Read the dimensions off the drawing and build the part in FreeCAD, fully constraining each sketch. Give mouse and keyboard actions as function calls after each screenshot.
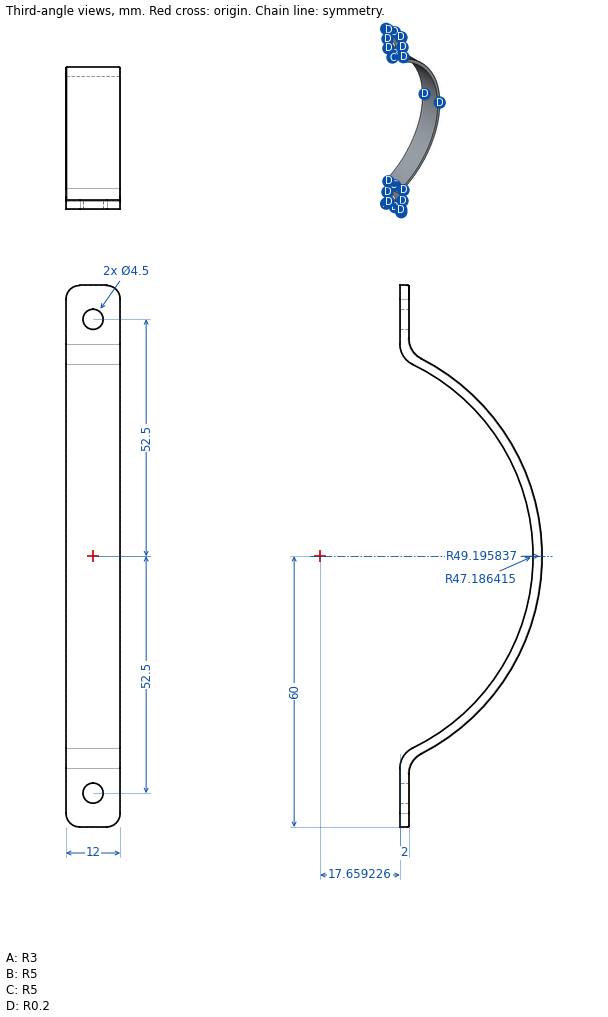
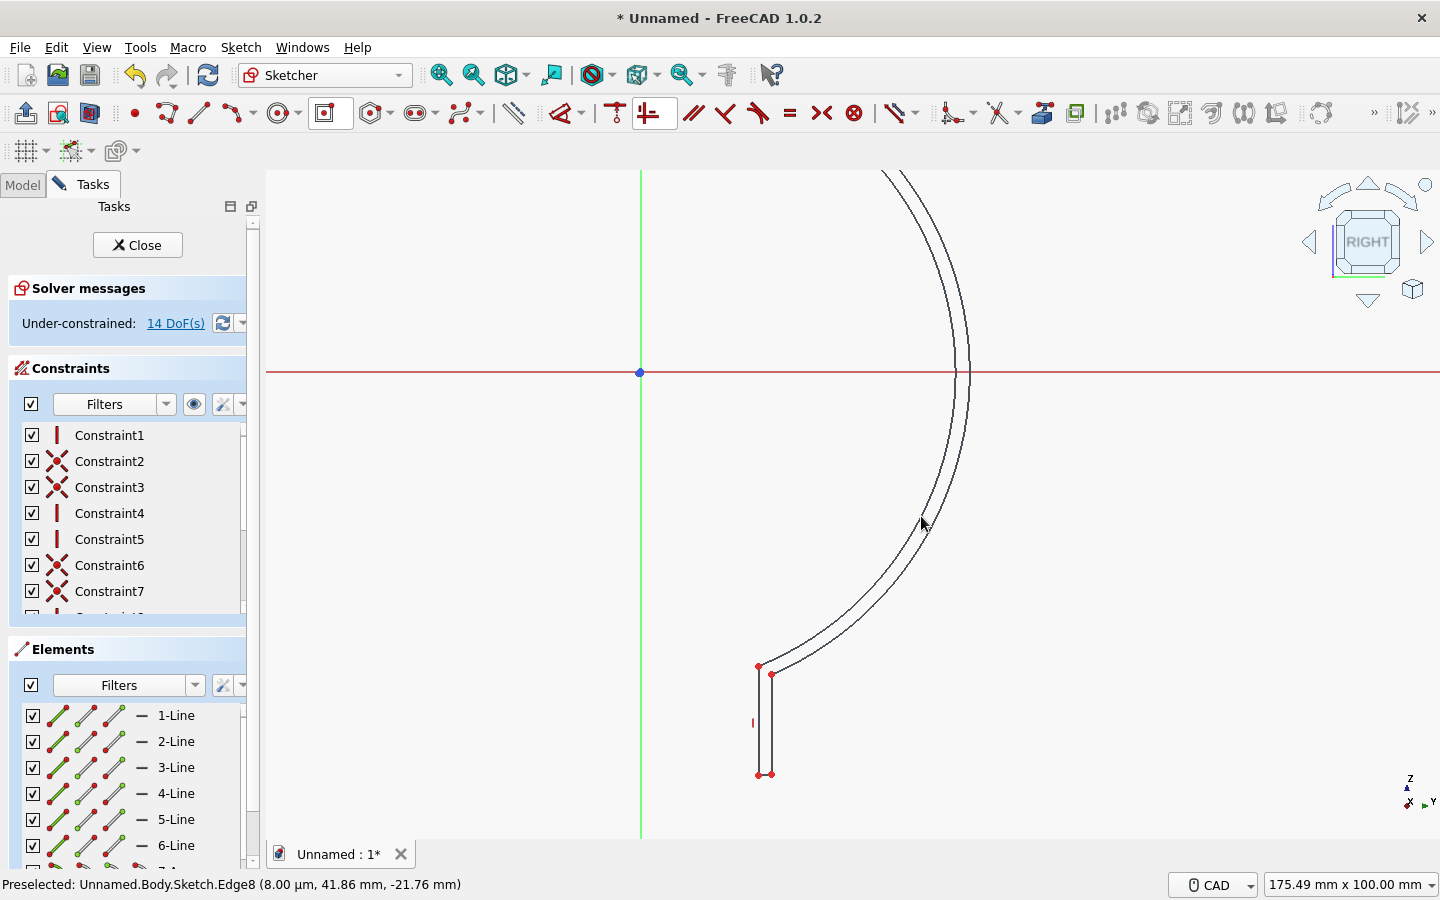
scroll(765, 775, up, 4)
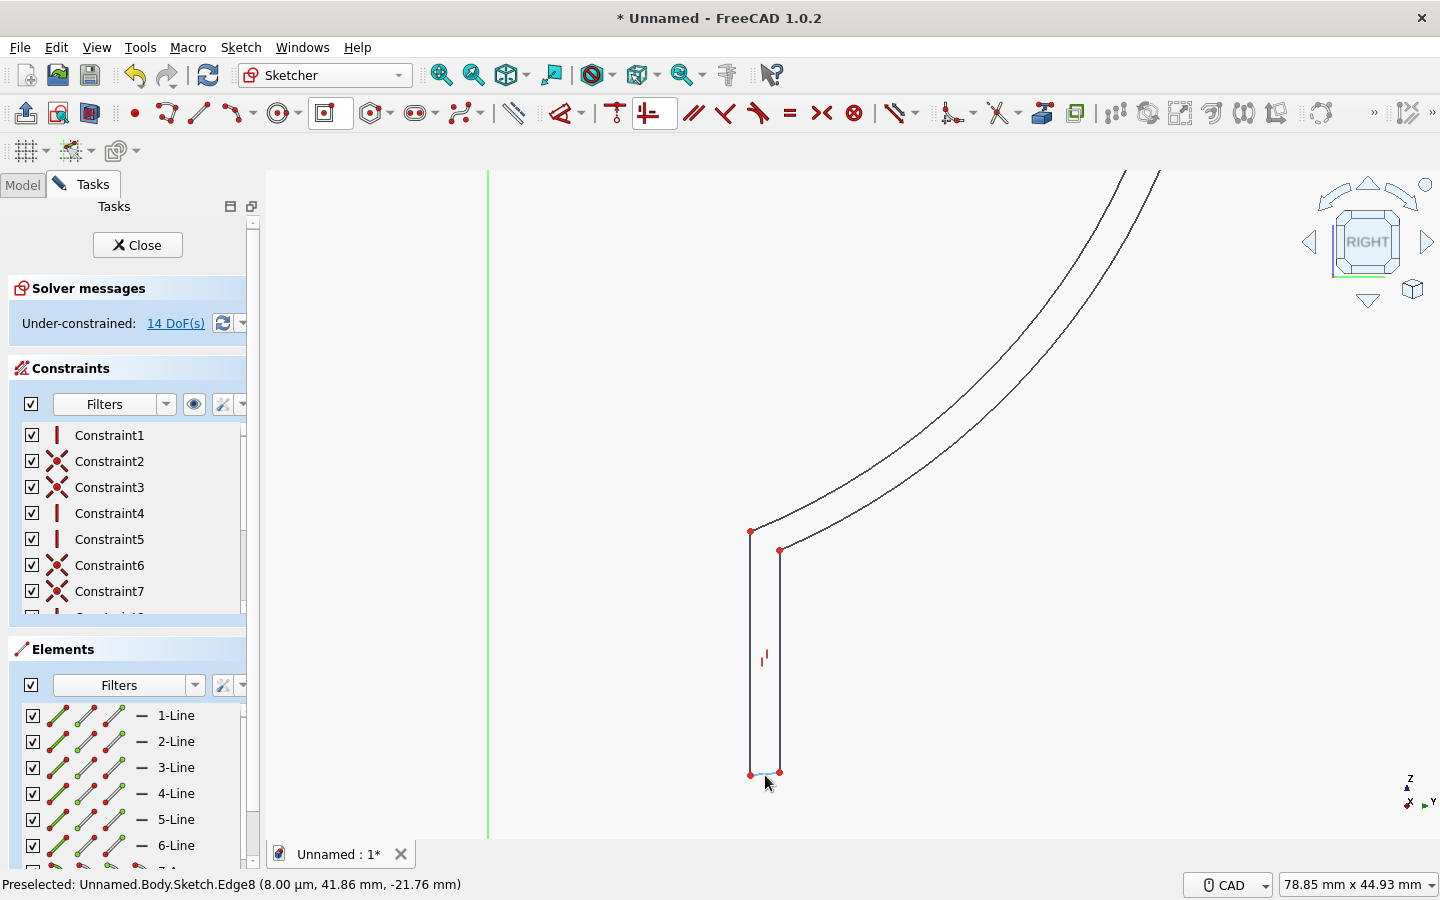
click(765, 774)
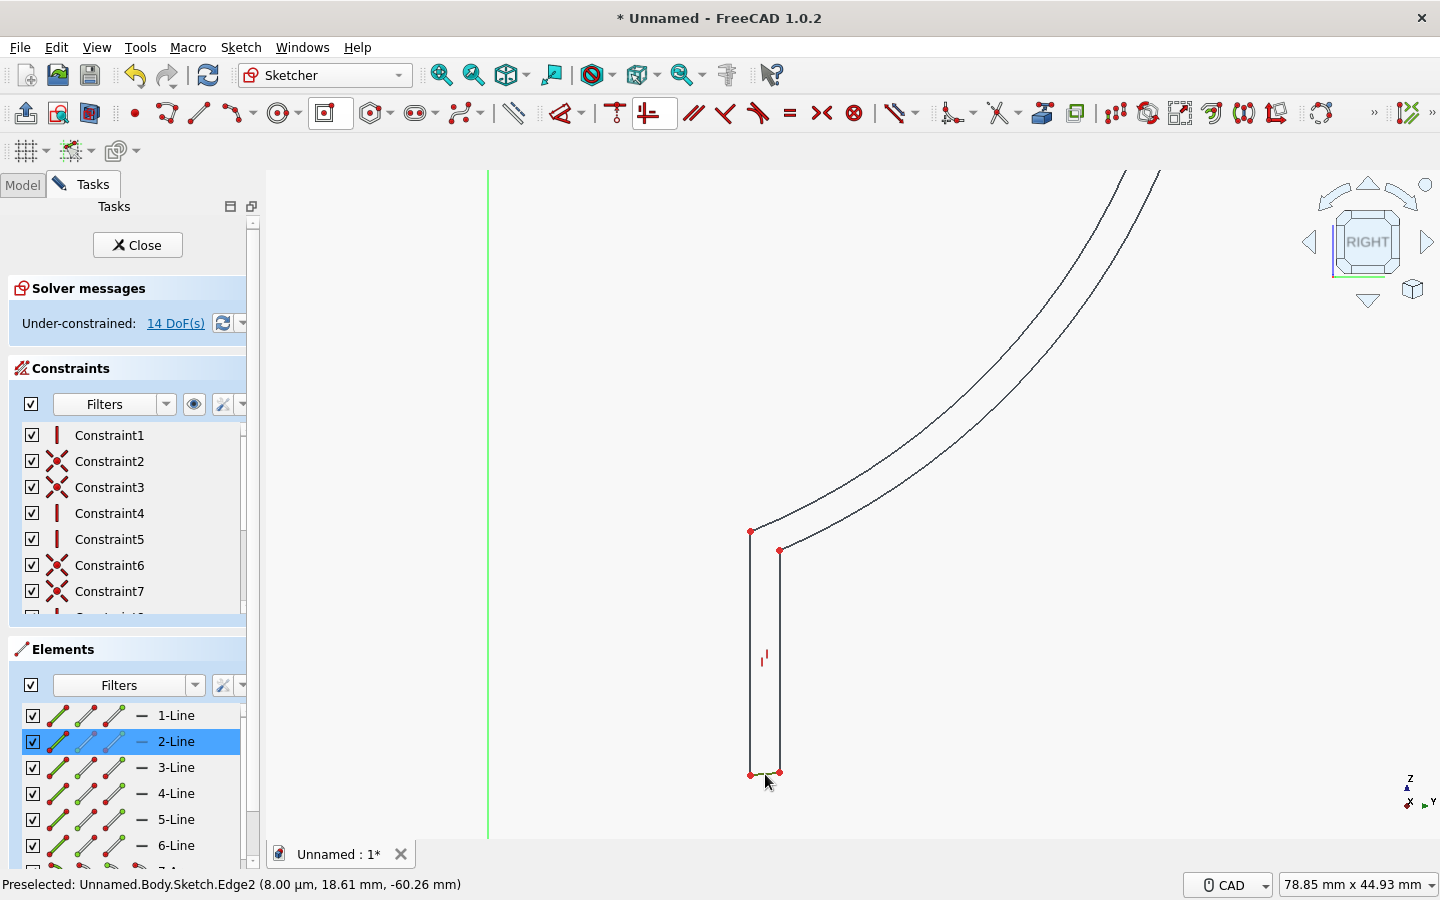
click(672, 114)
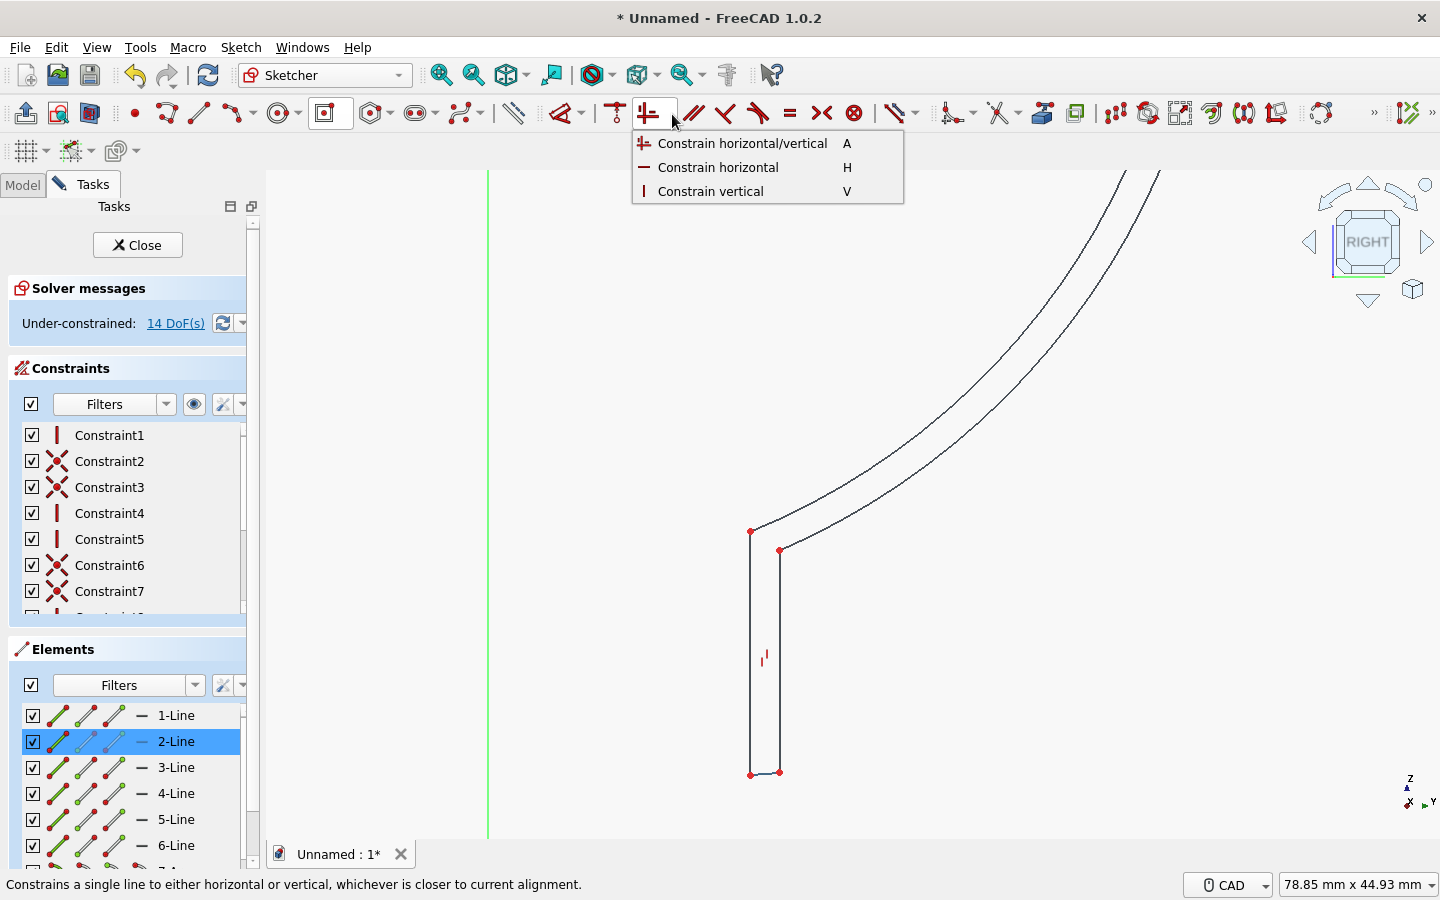
click(768, 167)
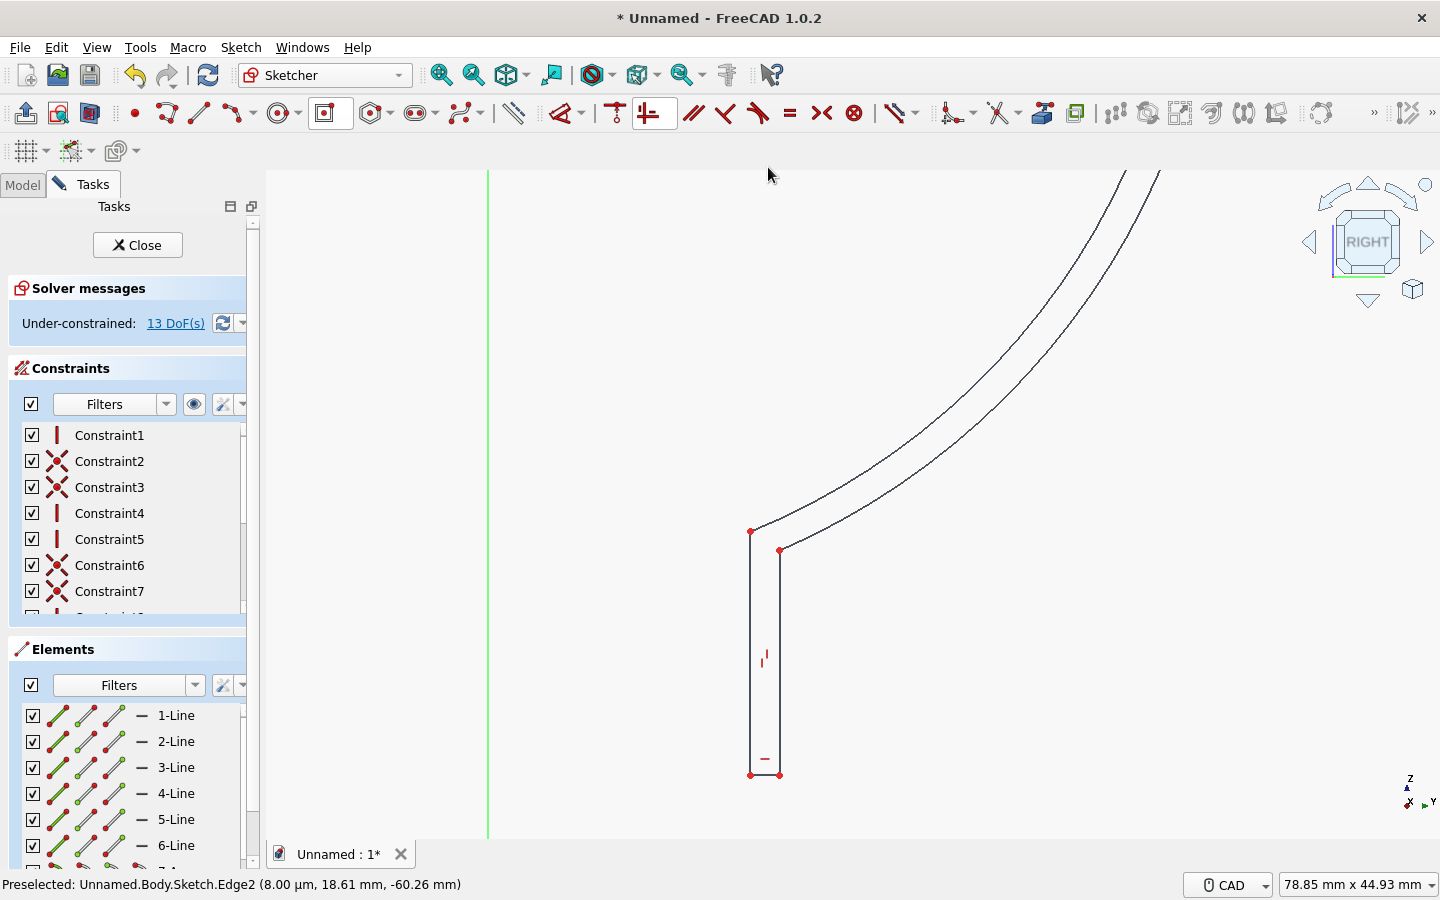
scroll(762, 710, down, 7)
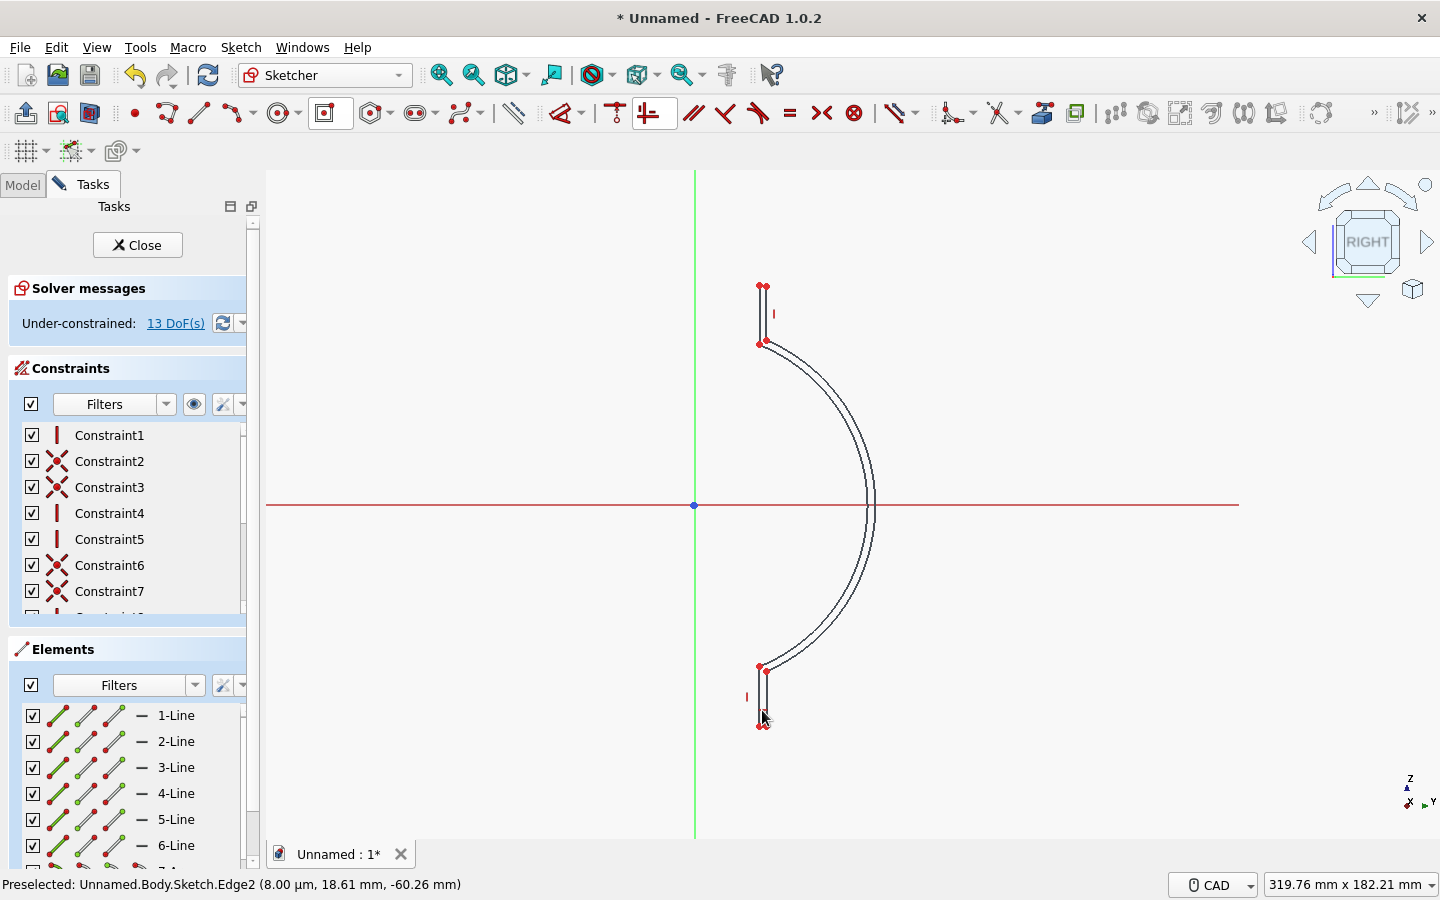
scroll(764, 286, up, 9)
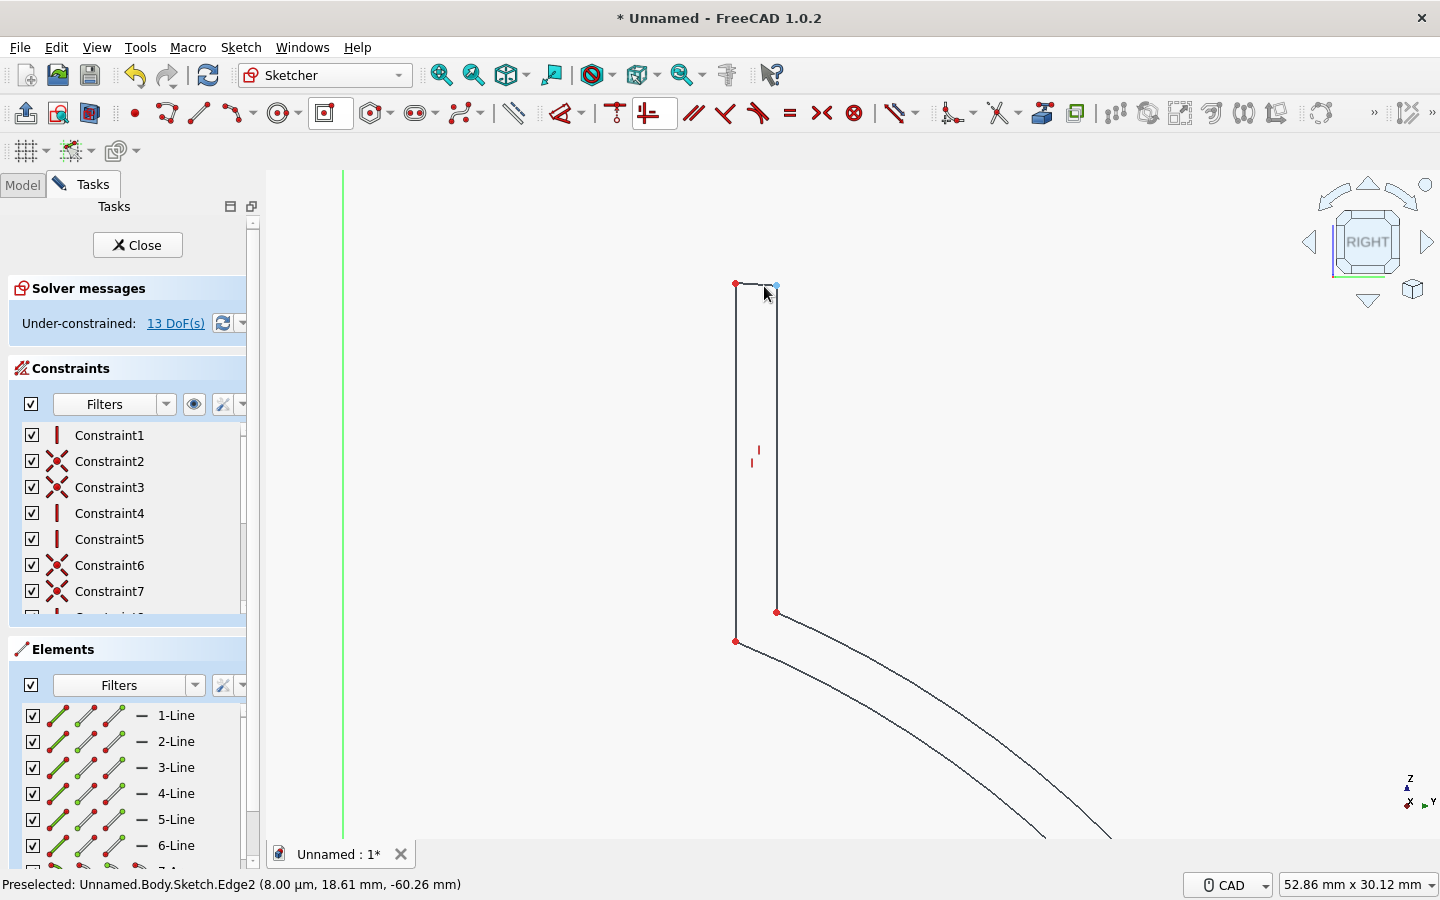
click(760, 285)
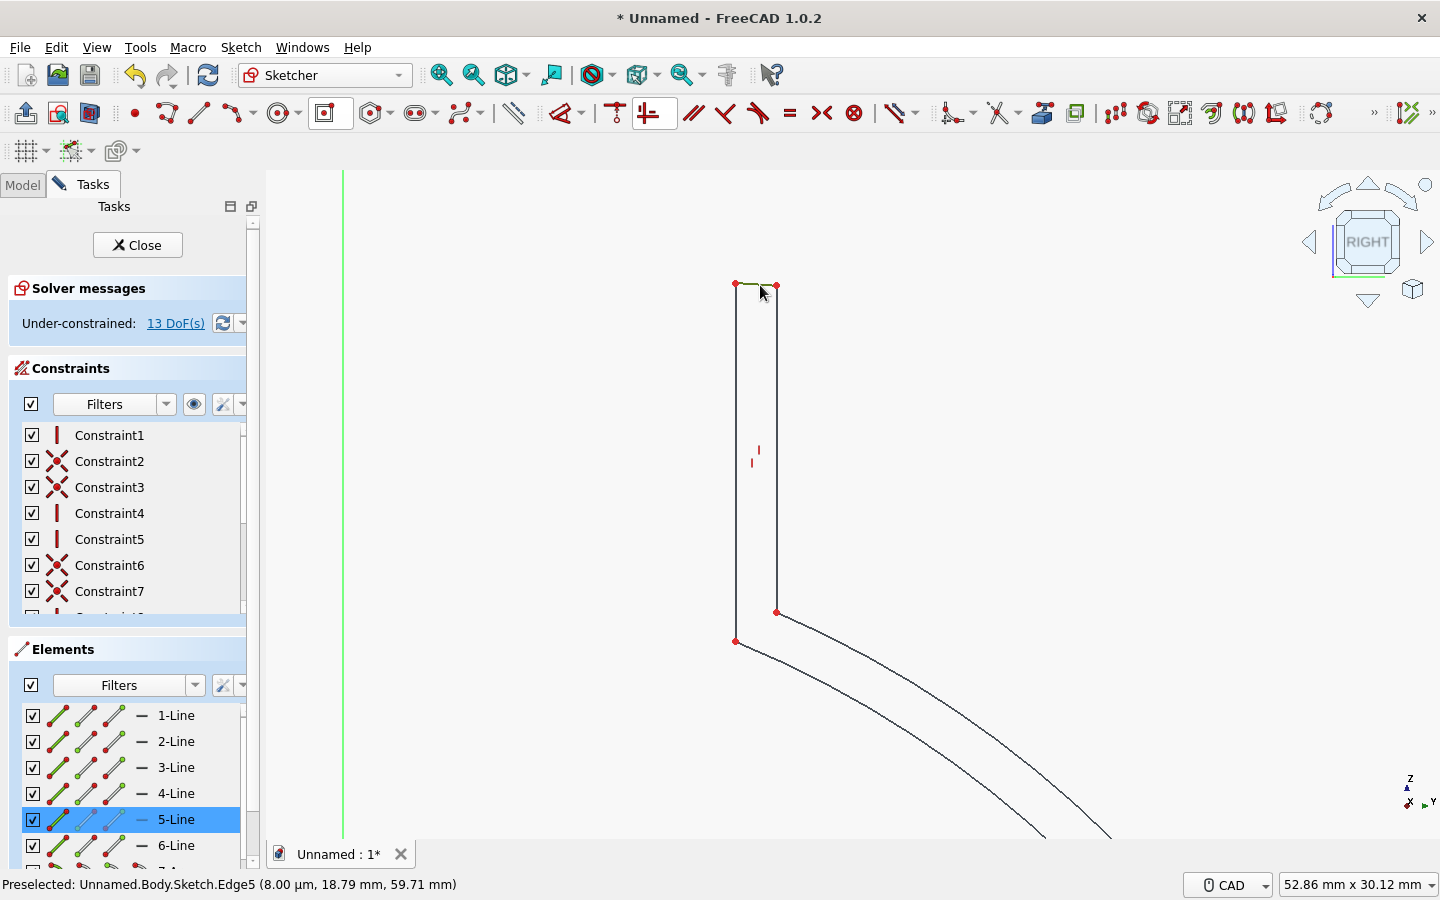
key(h)